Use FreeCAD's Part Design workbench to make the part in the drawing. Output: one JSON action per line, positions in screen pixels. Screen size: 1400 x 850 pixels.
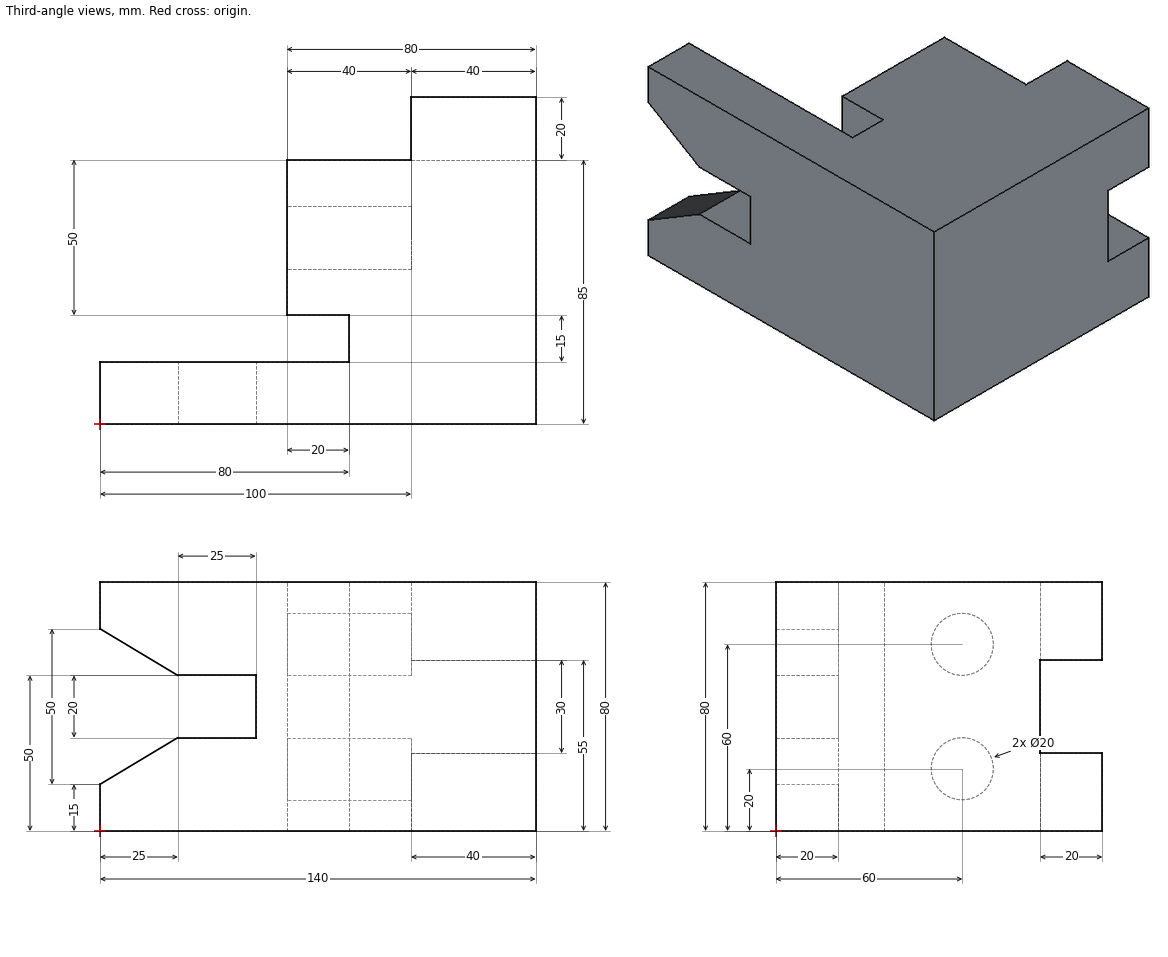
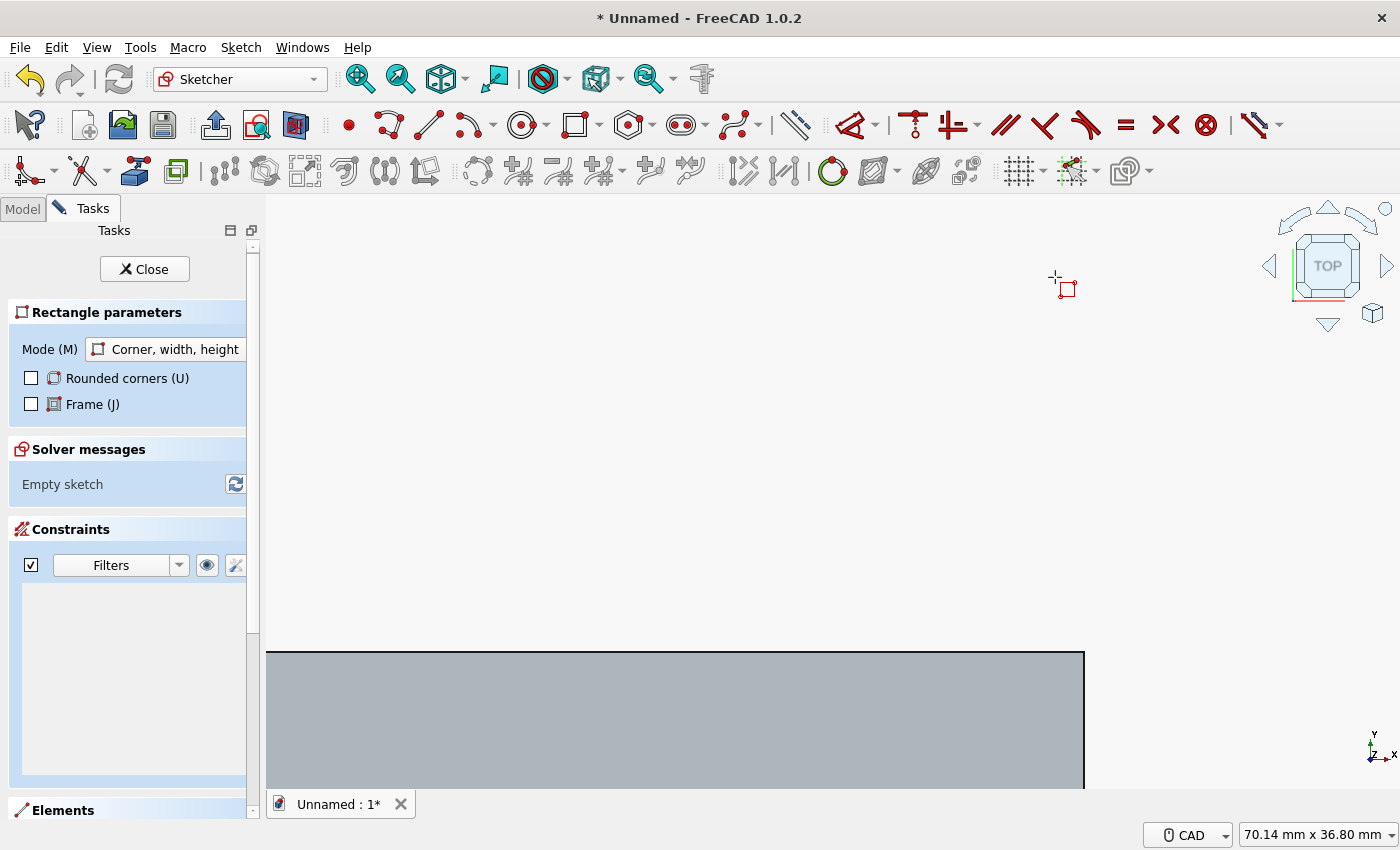
{"action": "left_click", "coordinate": [438, 328]}
{"action": "mouse_move", "coordinate": [1084, 652]}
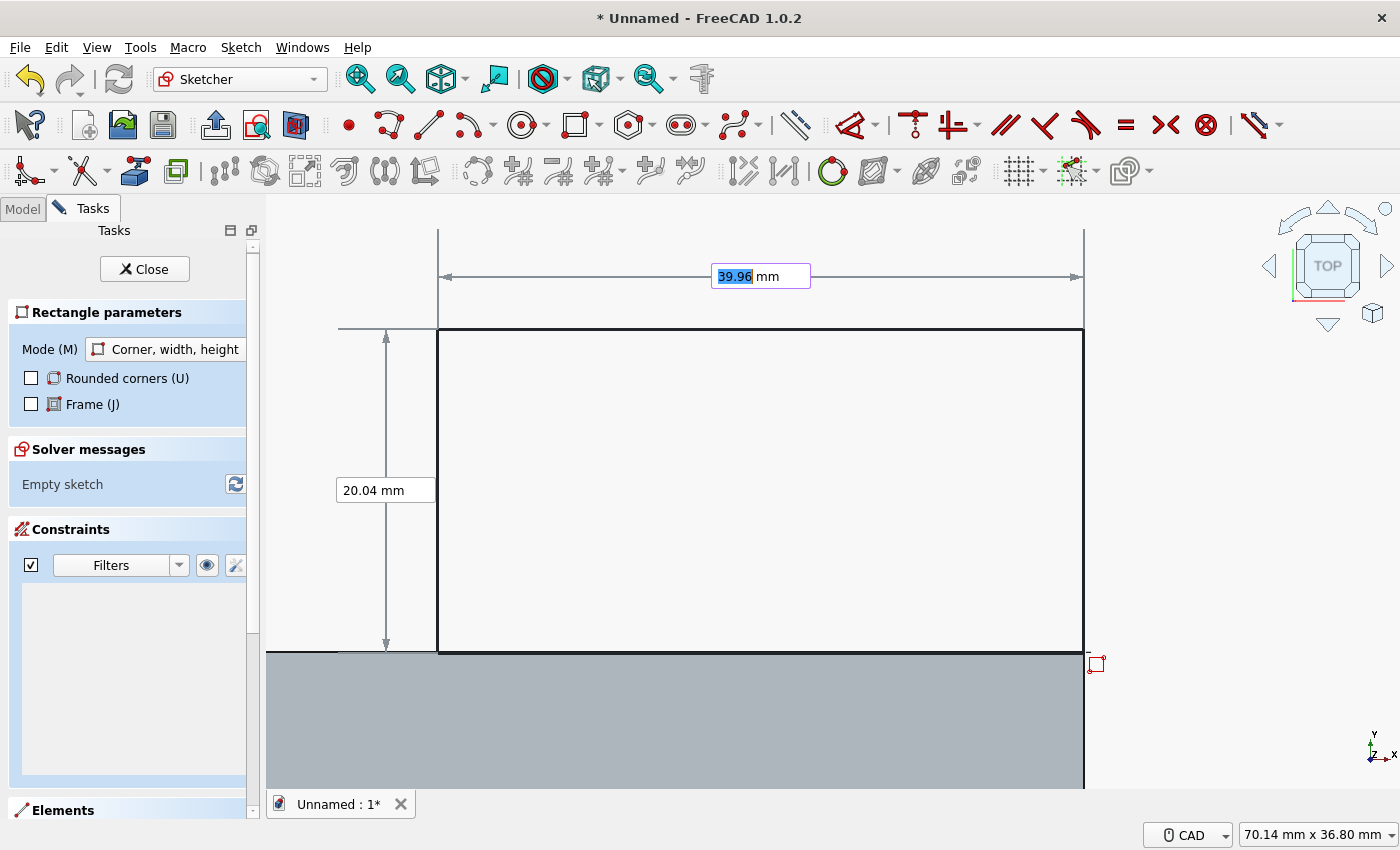
{"action": "type", "text": "40"}
{"action": "key", "text": "Tab"}
{"action": "type", "text": "20"}
{"action": "key", "text": "Return"}
{"action": "key", "text": "Escape"}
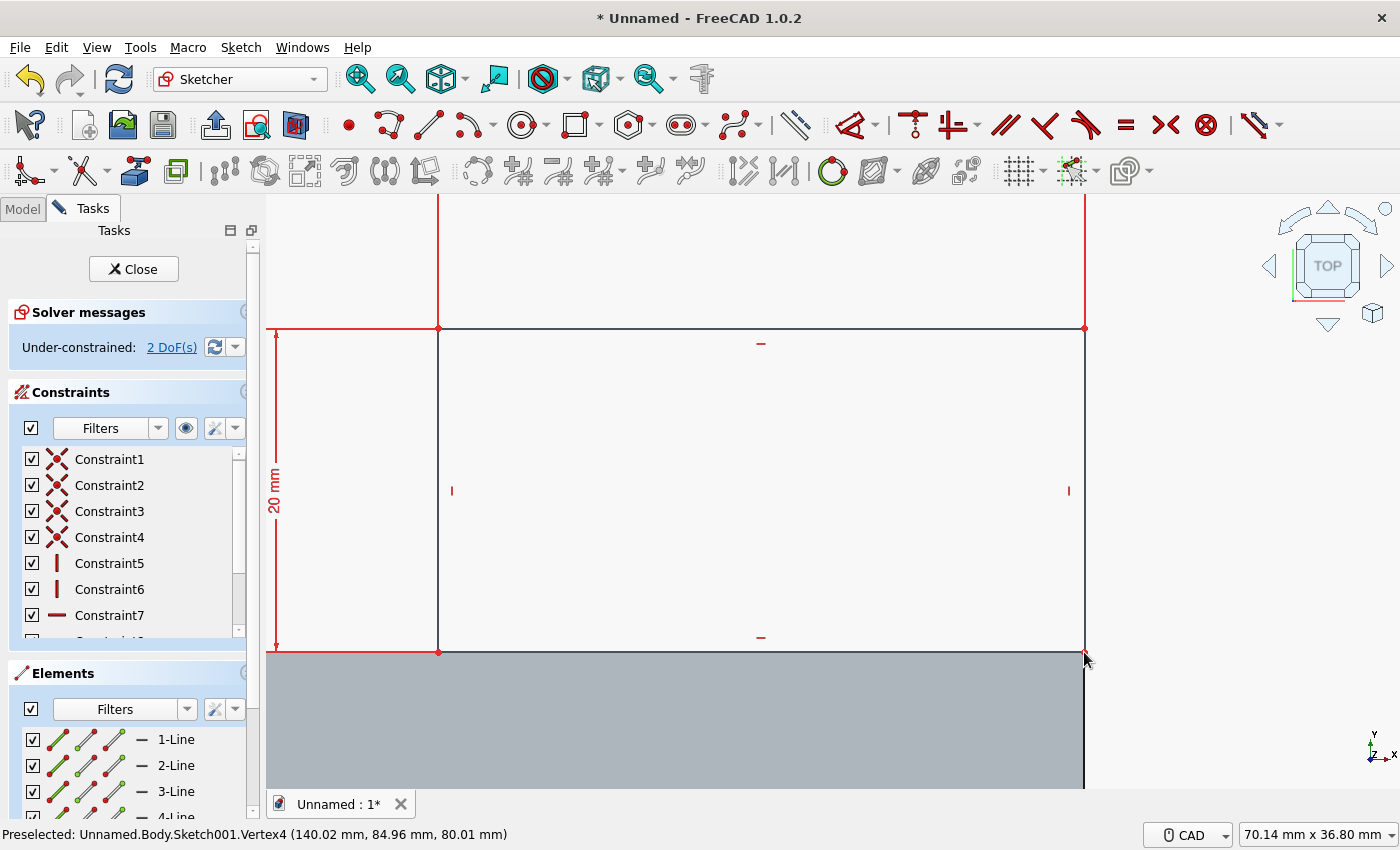
{"action": "key", "text": "d"}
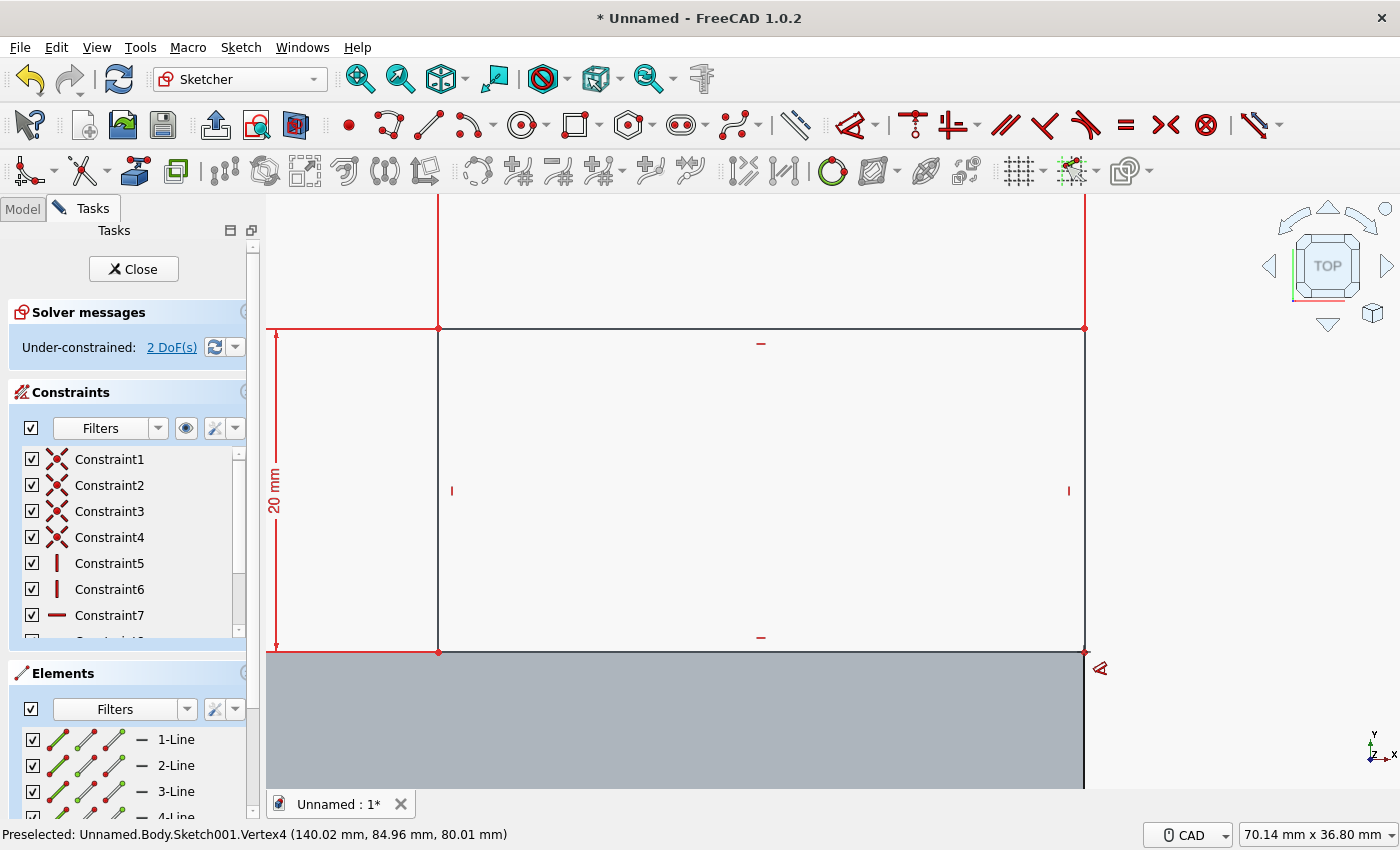
{"action": "left_click", "coordinate": [438, 652]}
{"action": "left_click", "coordinate": [472, 707]}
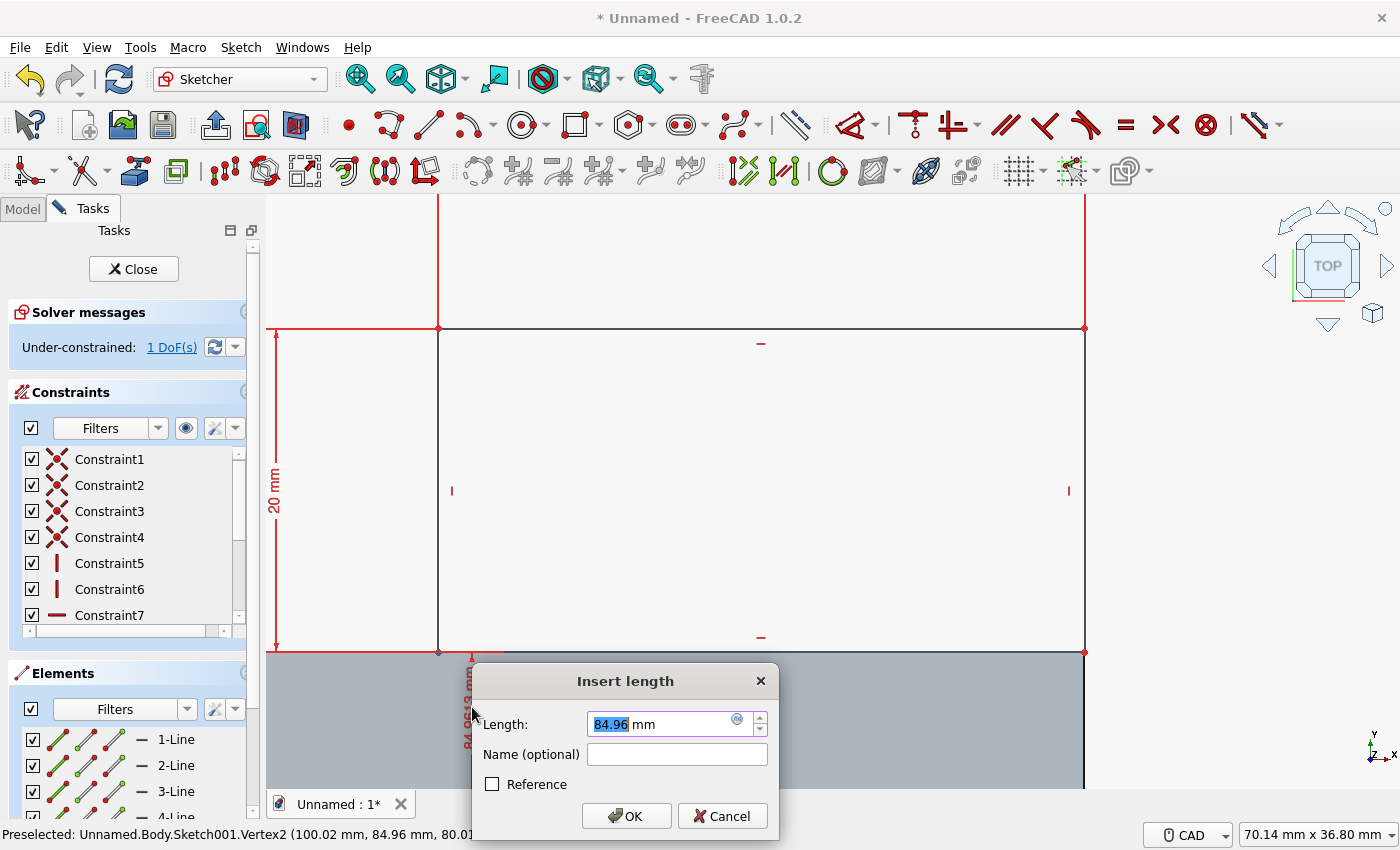
{"action": "type", "text": "85"}
{"action": "key", "text": "Return"}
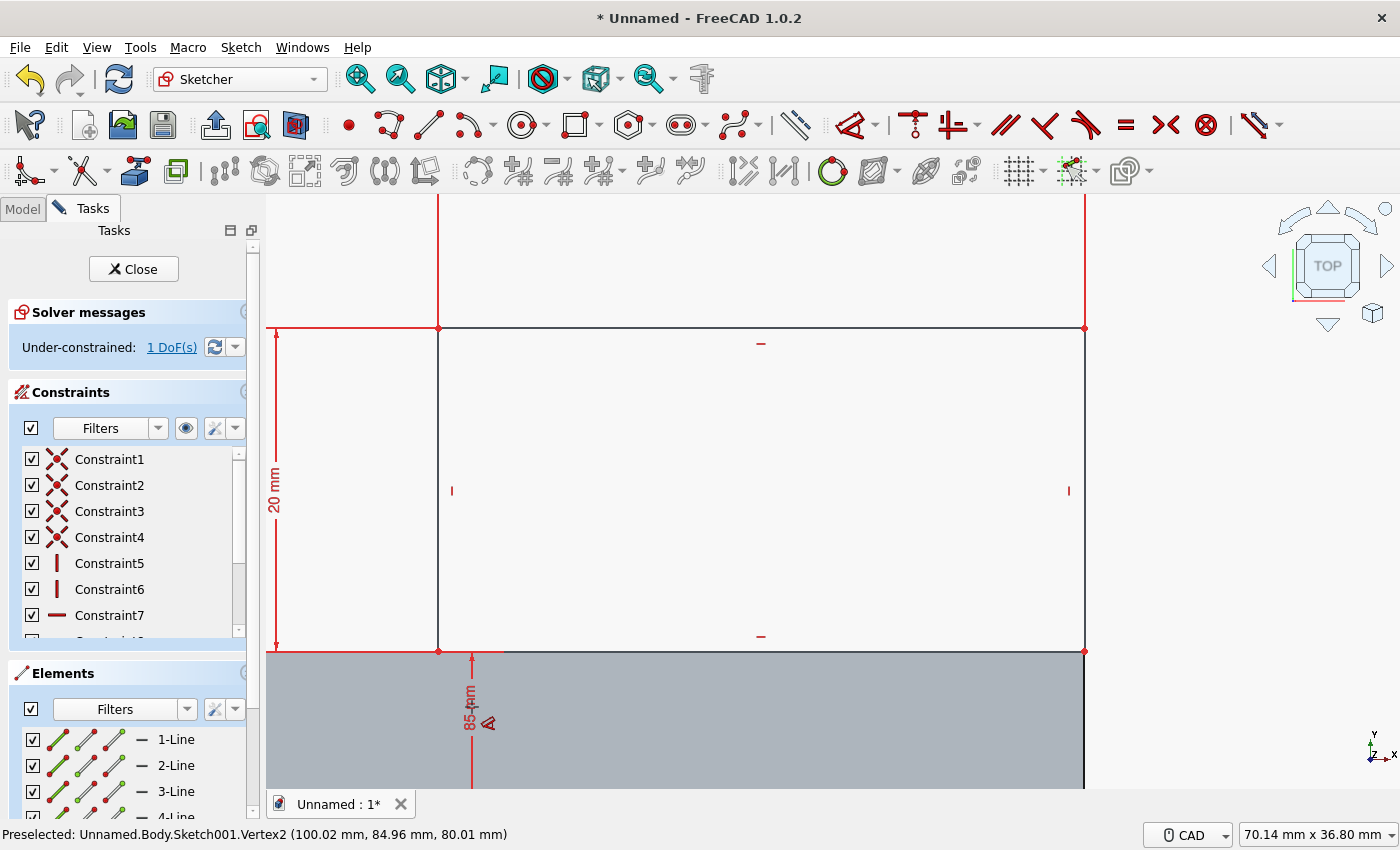
{"action": "left_click", "coordinate": [438, 328]}
{"action": "left_click", "coordinate": [366, 294]}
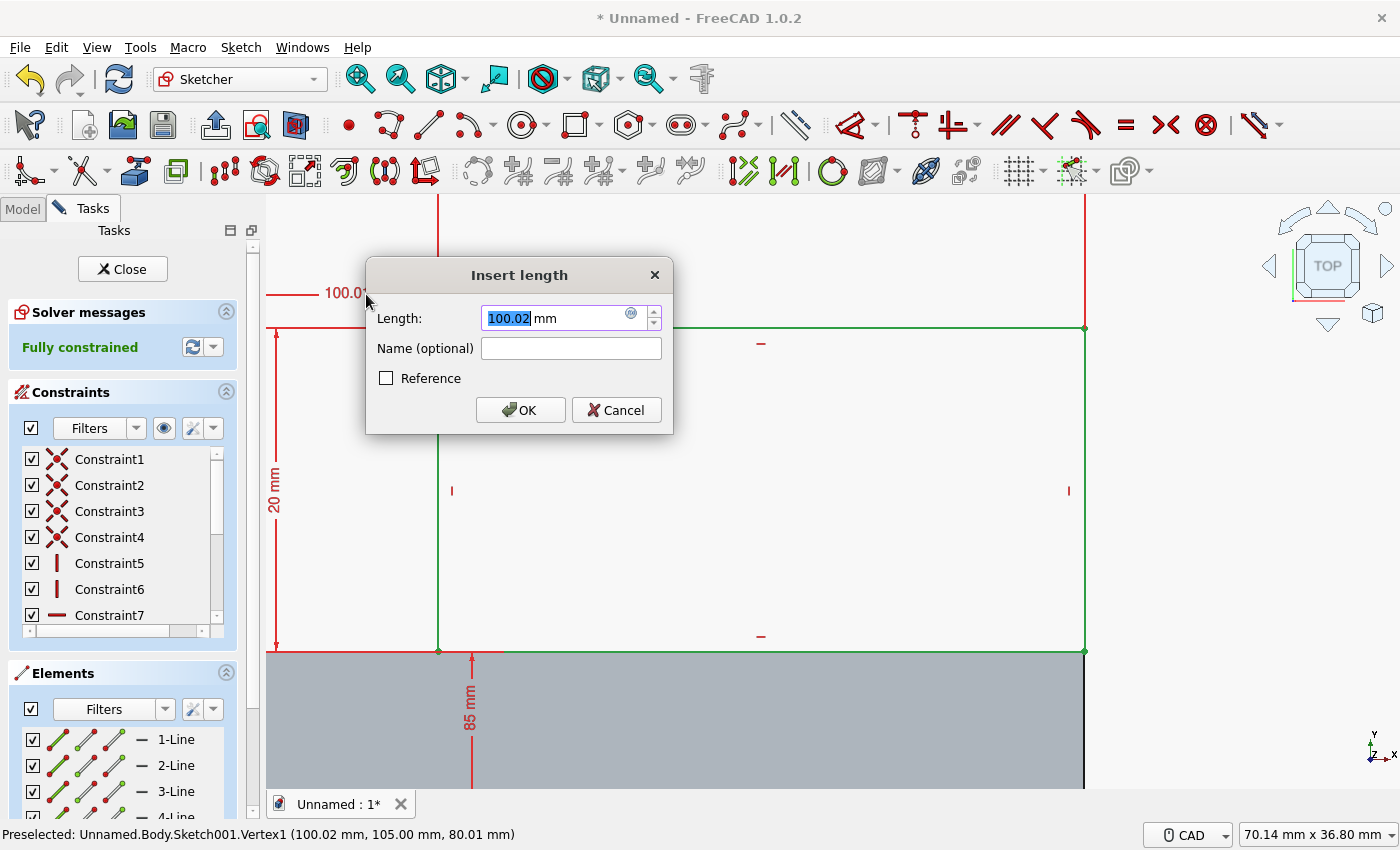
{"action": "type", "text": "100"}
{"action": "key", "text": "Return"}
{"action": "key", "text": "Escape"}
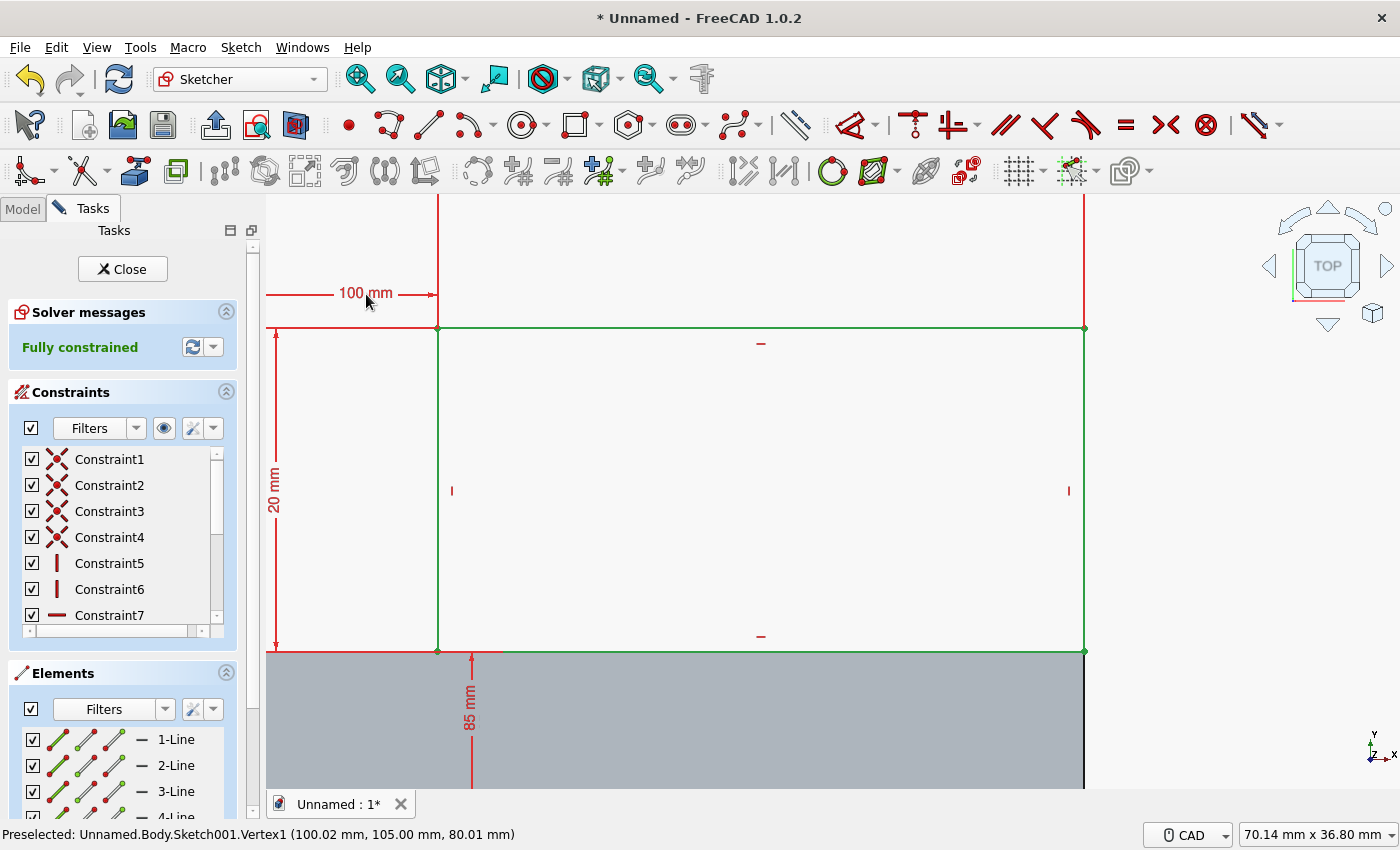
{"action": "left_click", "coordinate": [123, 269]}